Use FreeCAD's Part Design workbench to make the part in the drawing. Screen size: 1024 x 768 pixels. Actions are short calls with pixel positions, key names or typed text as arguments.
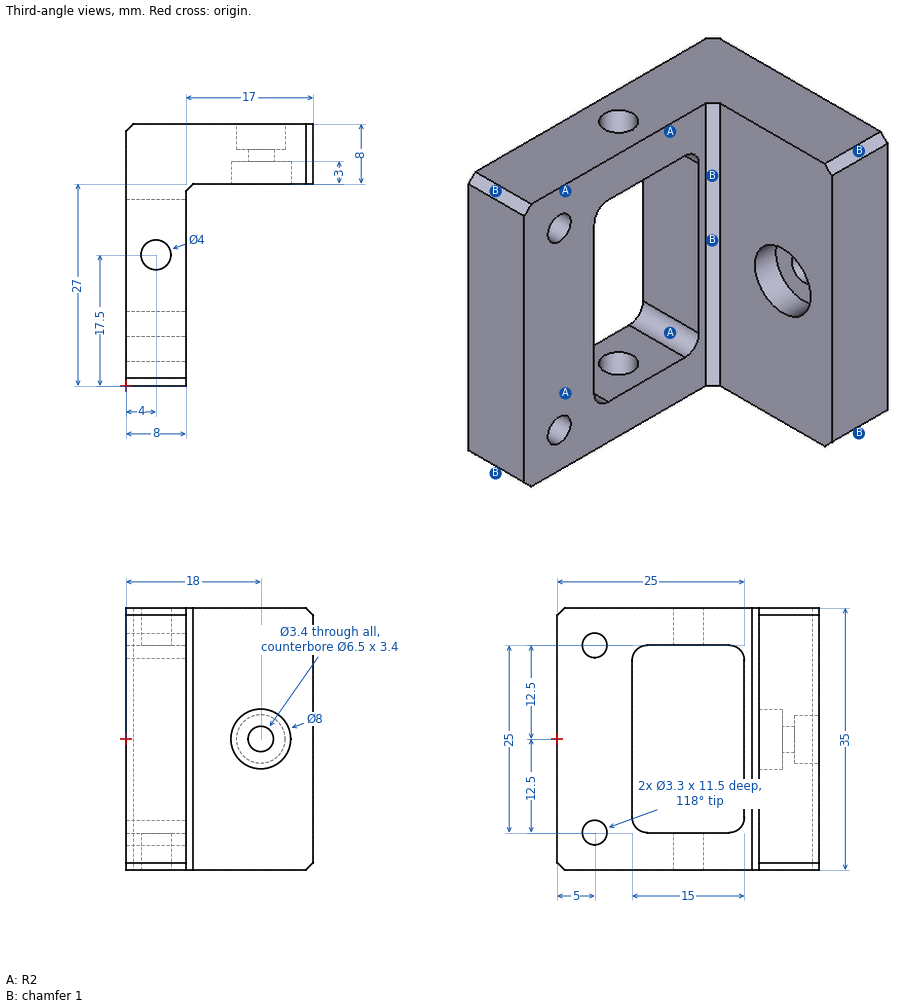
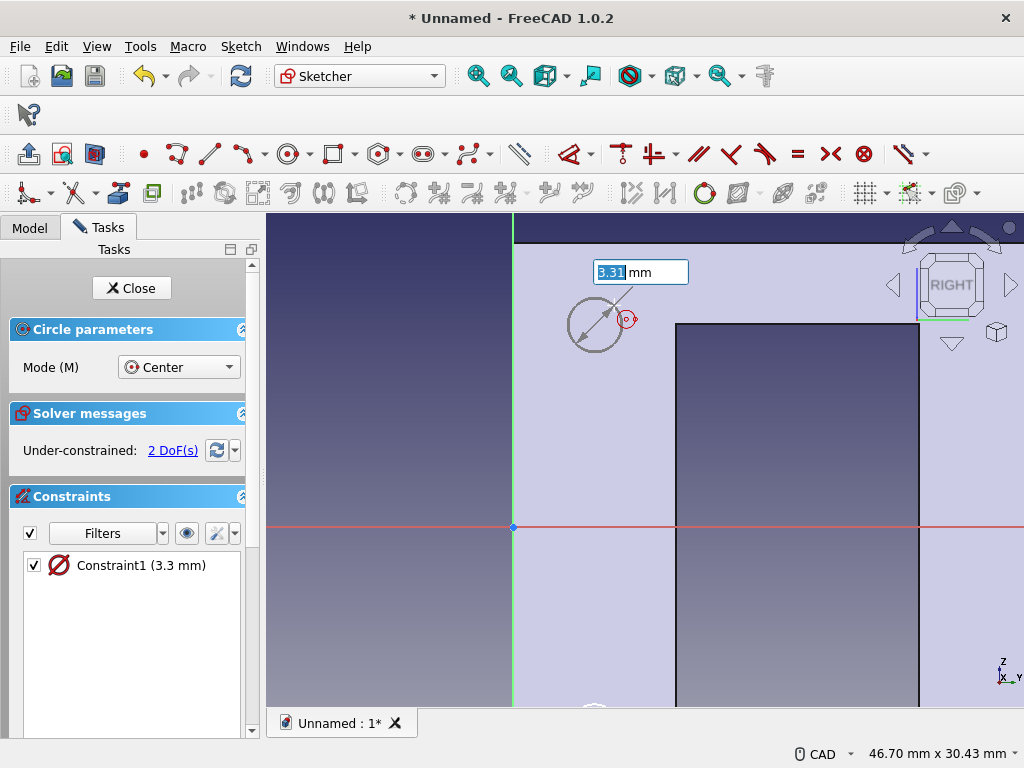
text(3.3)
key(Return)
key(Escape)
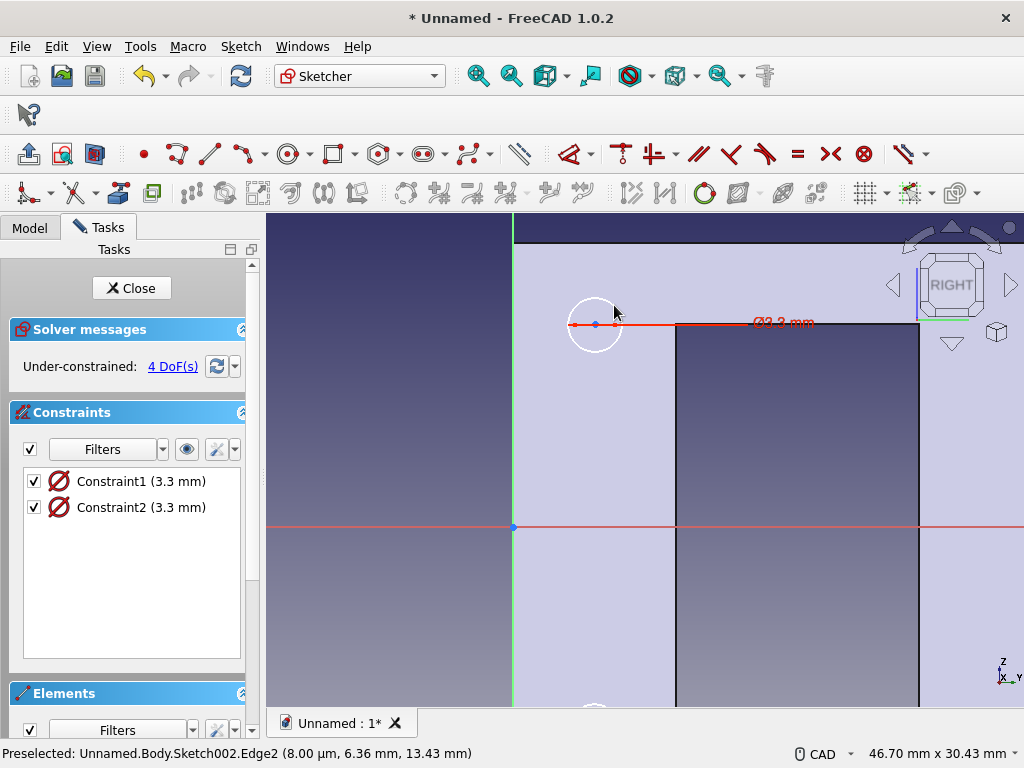
key(d)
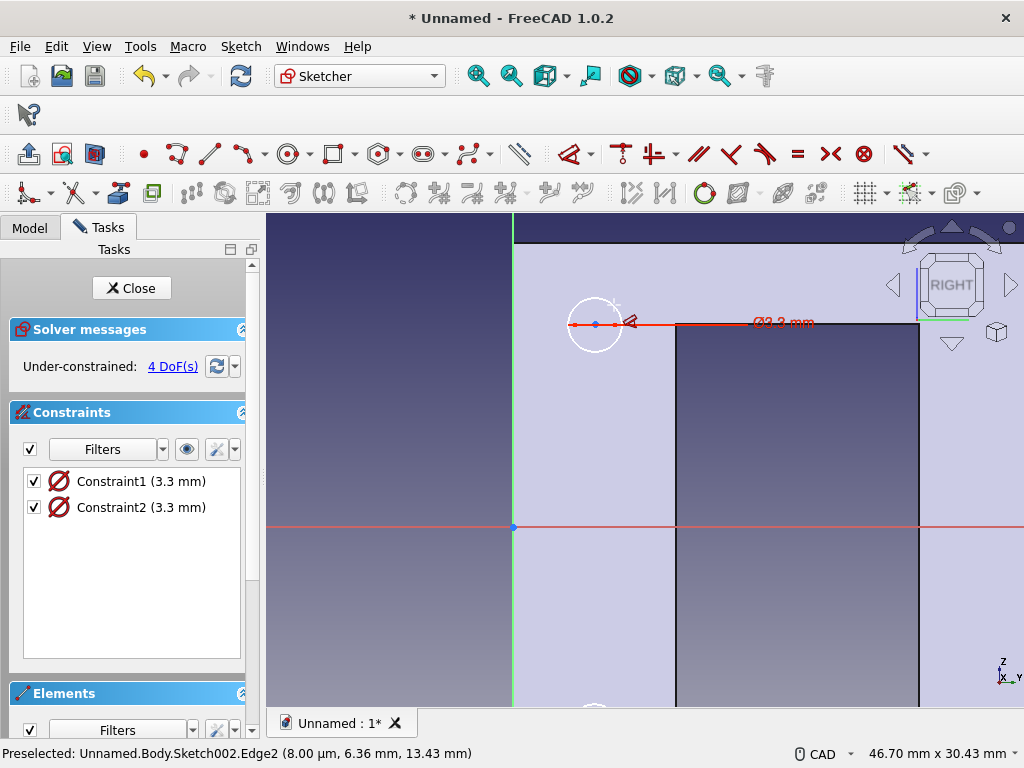
scroll(595, 323, down, 2)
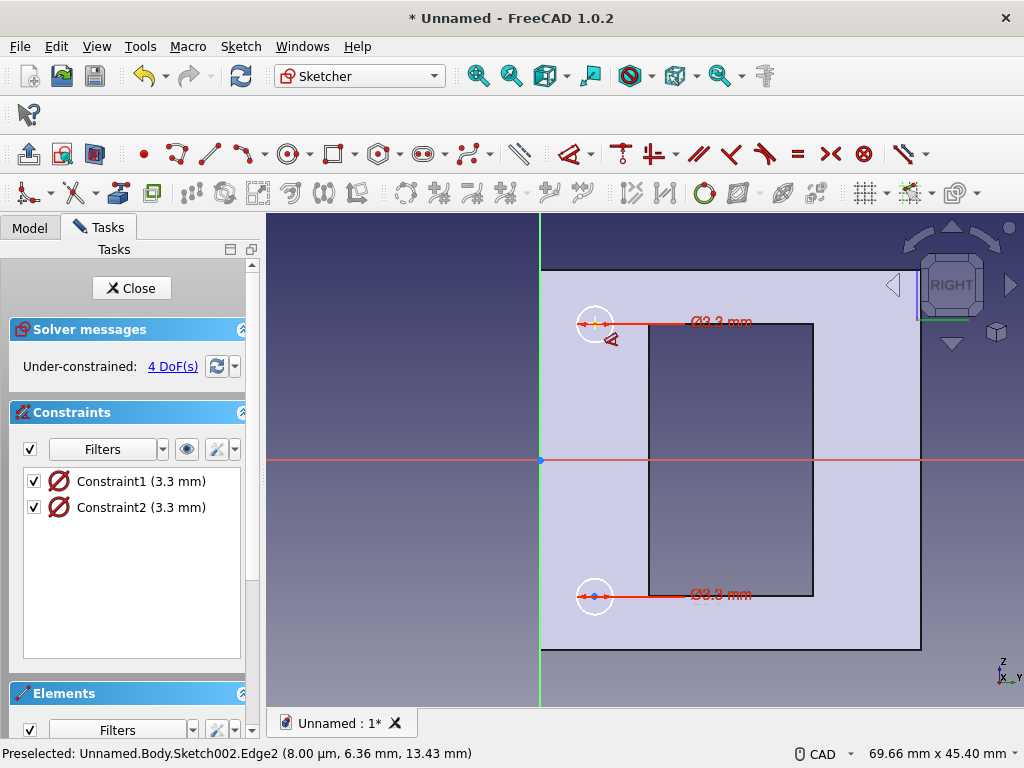
click(595, 597)
click(568, 631)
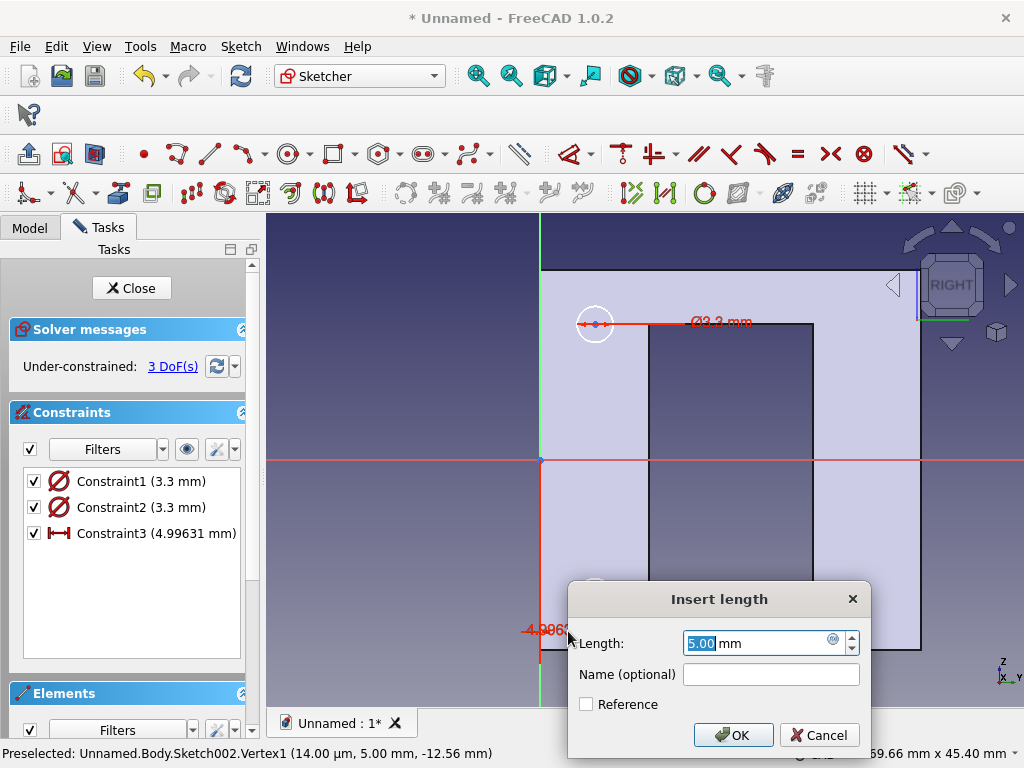
text(5)
key(Return)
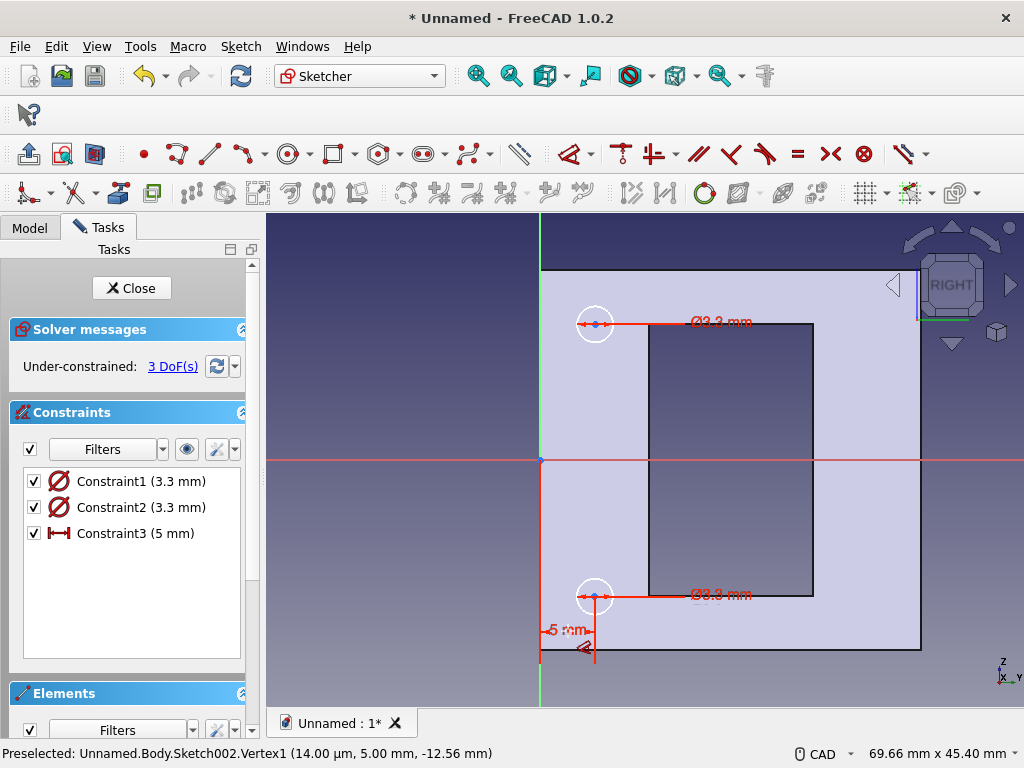
click(595, 324)
click(568, 290)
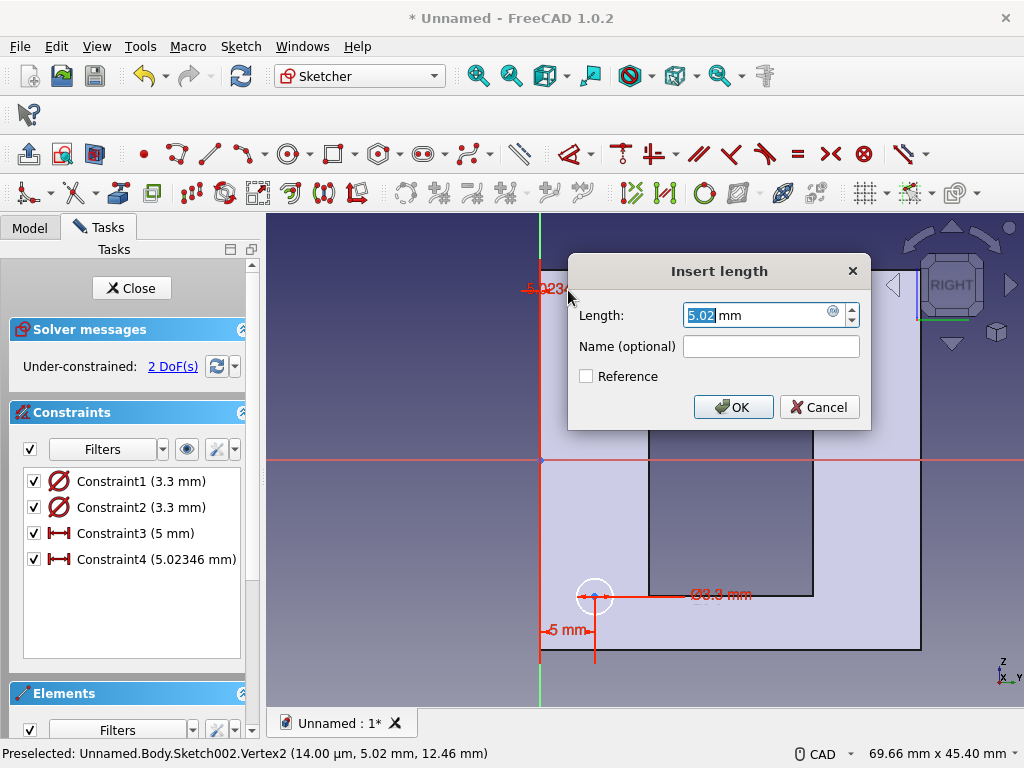
text(5)
key(Return)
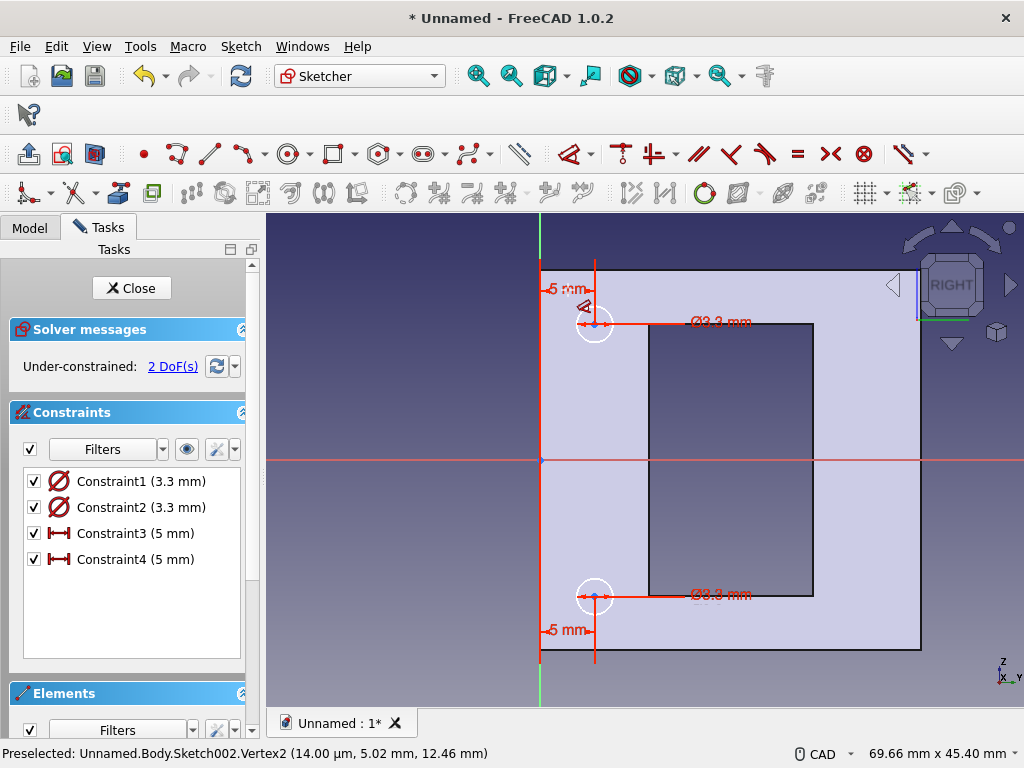
click(595, 597)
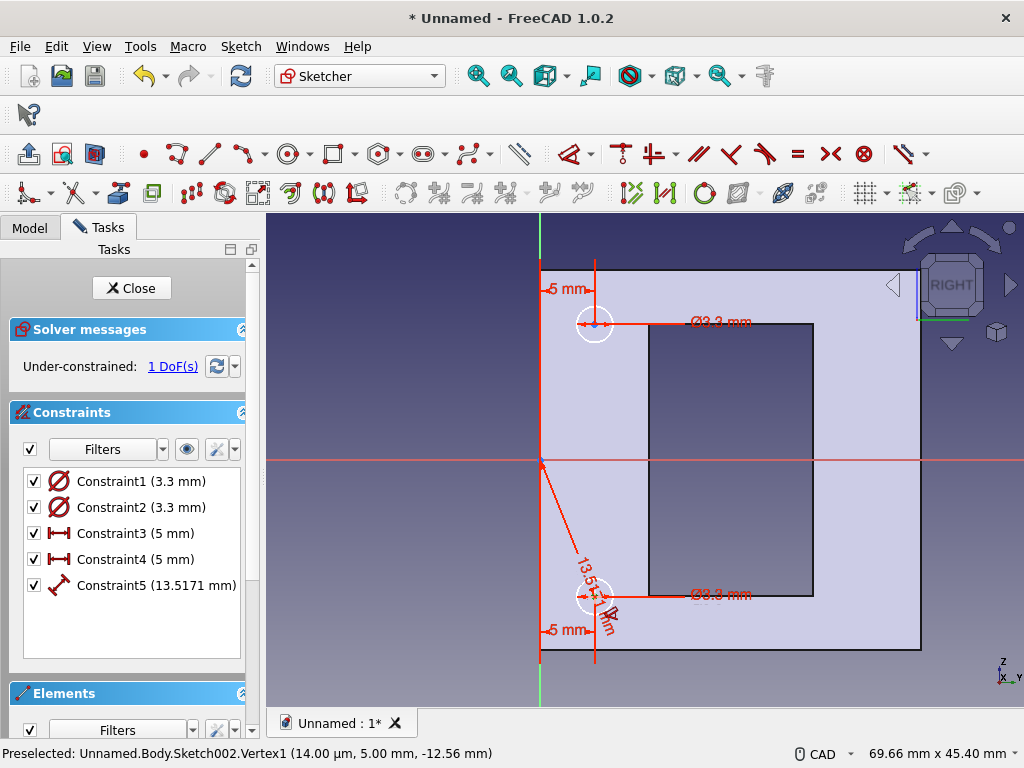
click(595, 324)
click(629, 398)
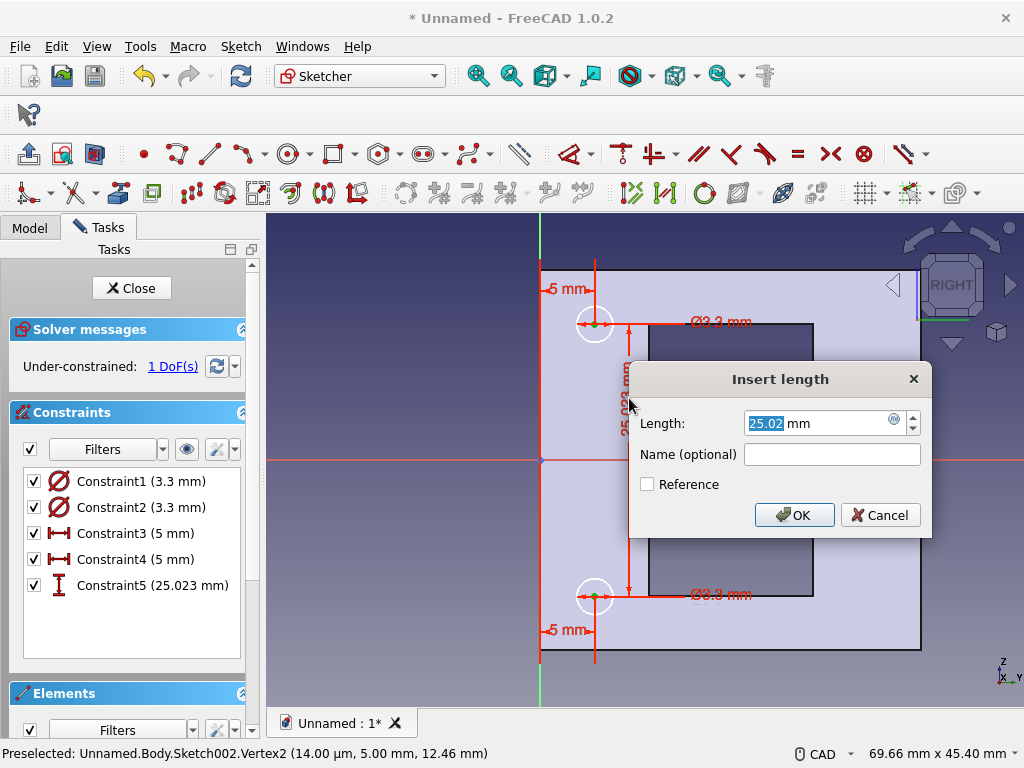
text(25)
key(Return)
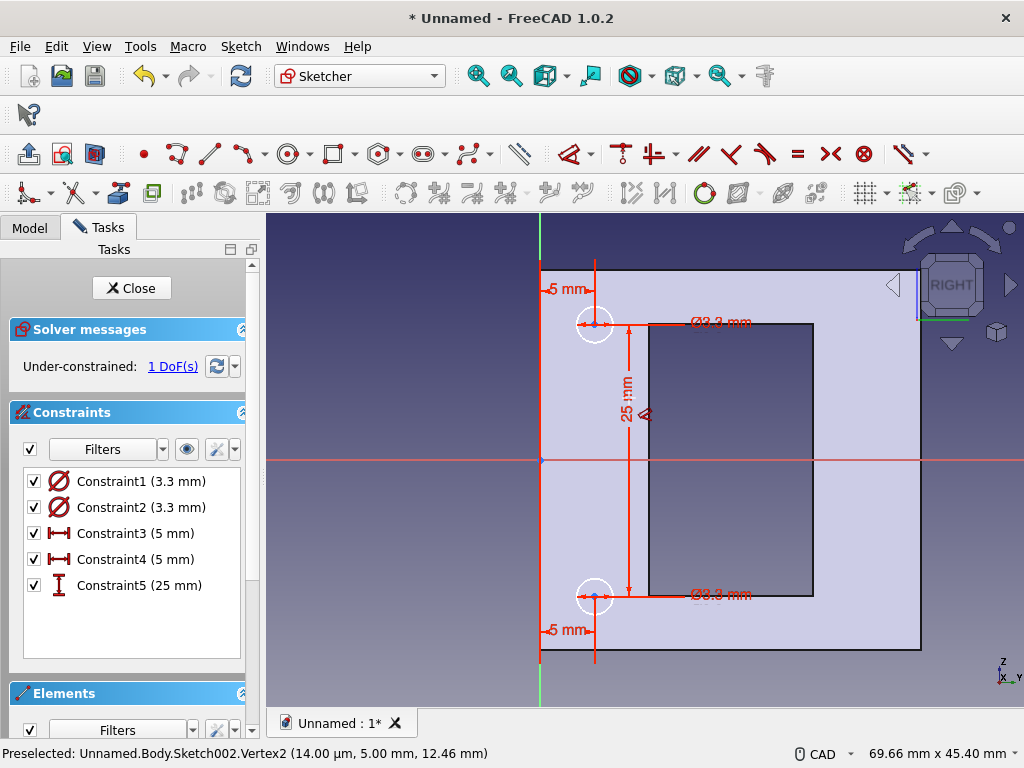
click(595, 597)
click(506, 528)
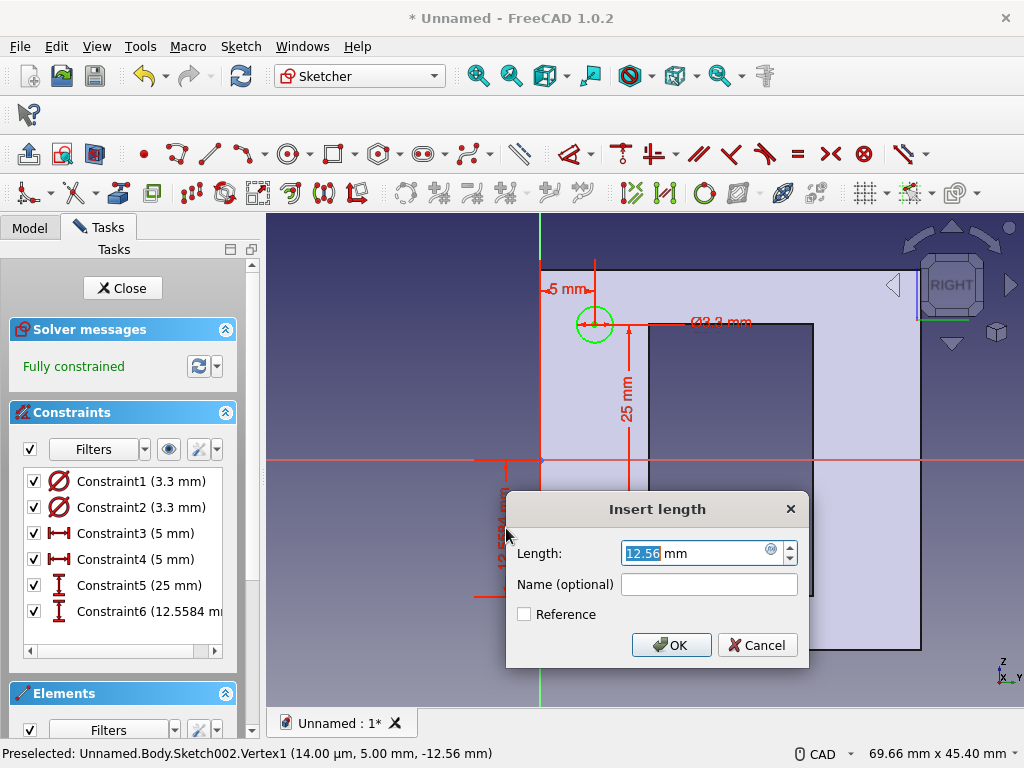
text(12.5)
key(Return)
key(Escape)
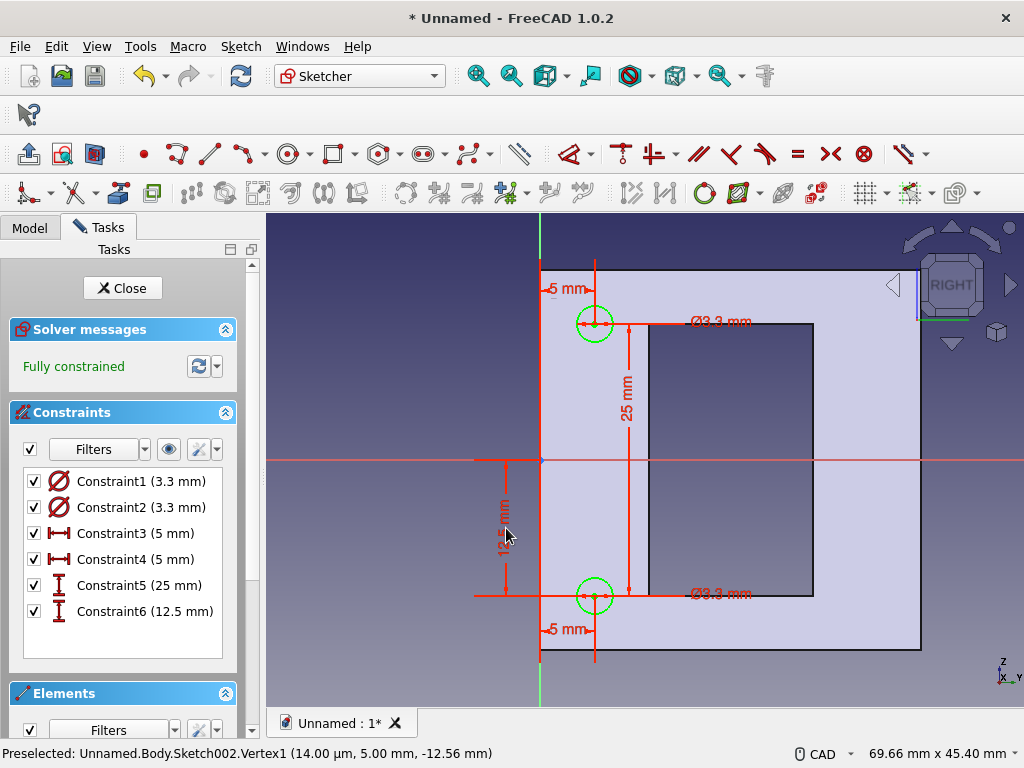
click(123, 288)